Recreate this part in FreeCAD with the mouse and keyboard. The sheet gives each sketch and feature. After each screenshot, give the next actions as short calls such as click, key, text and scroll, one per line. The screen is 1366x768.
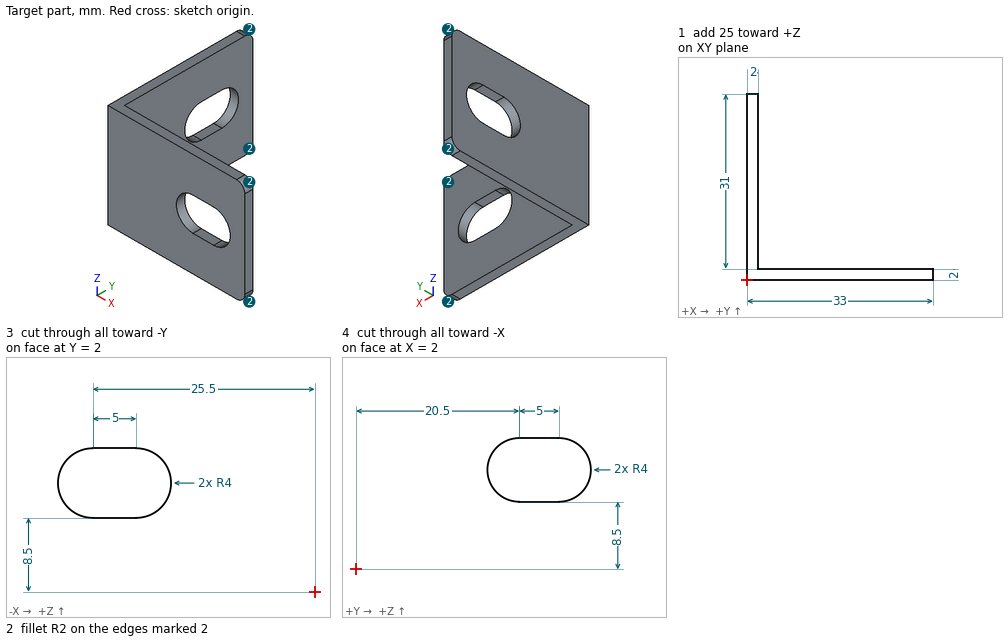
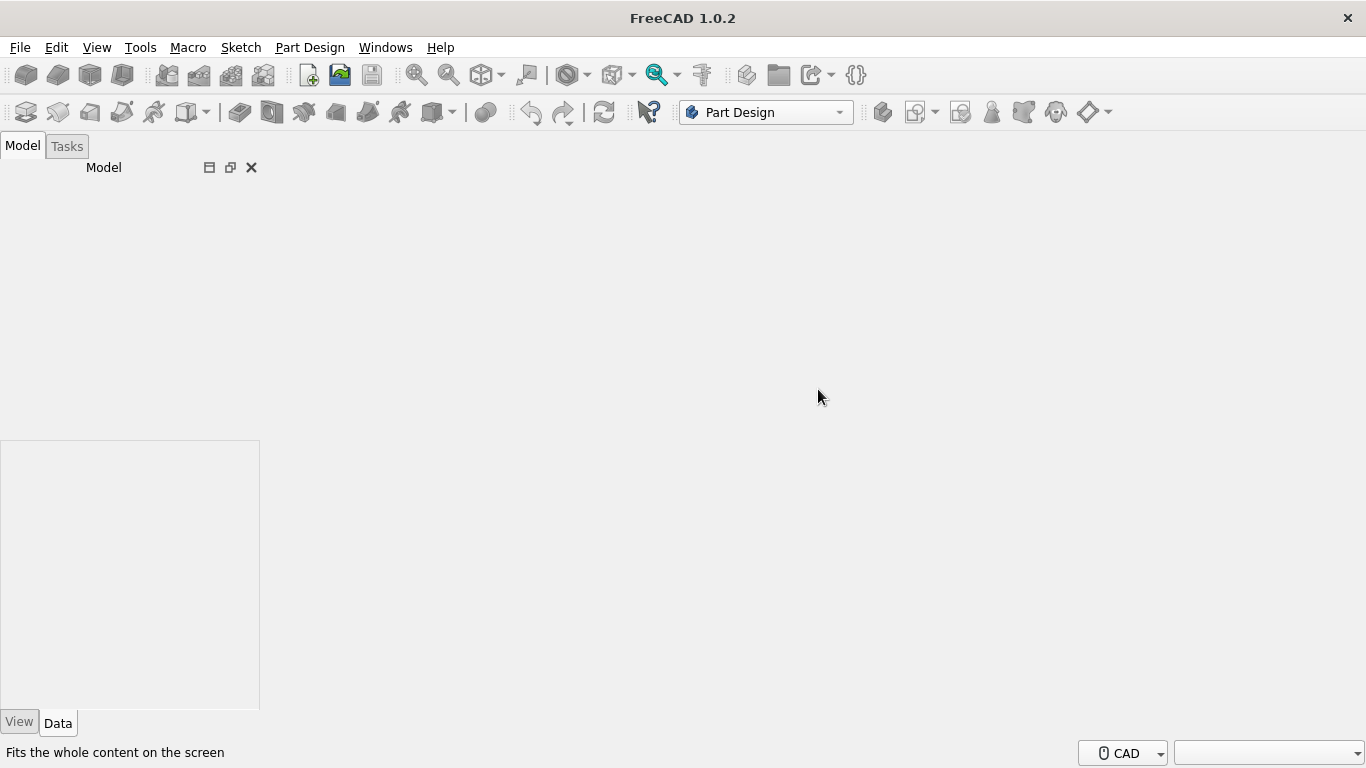
key(ctrl+n)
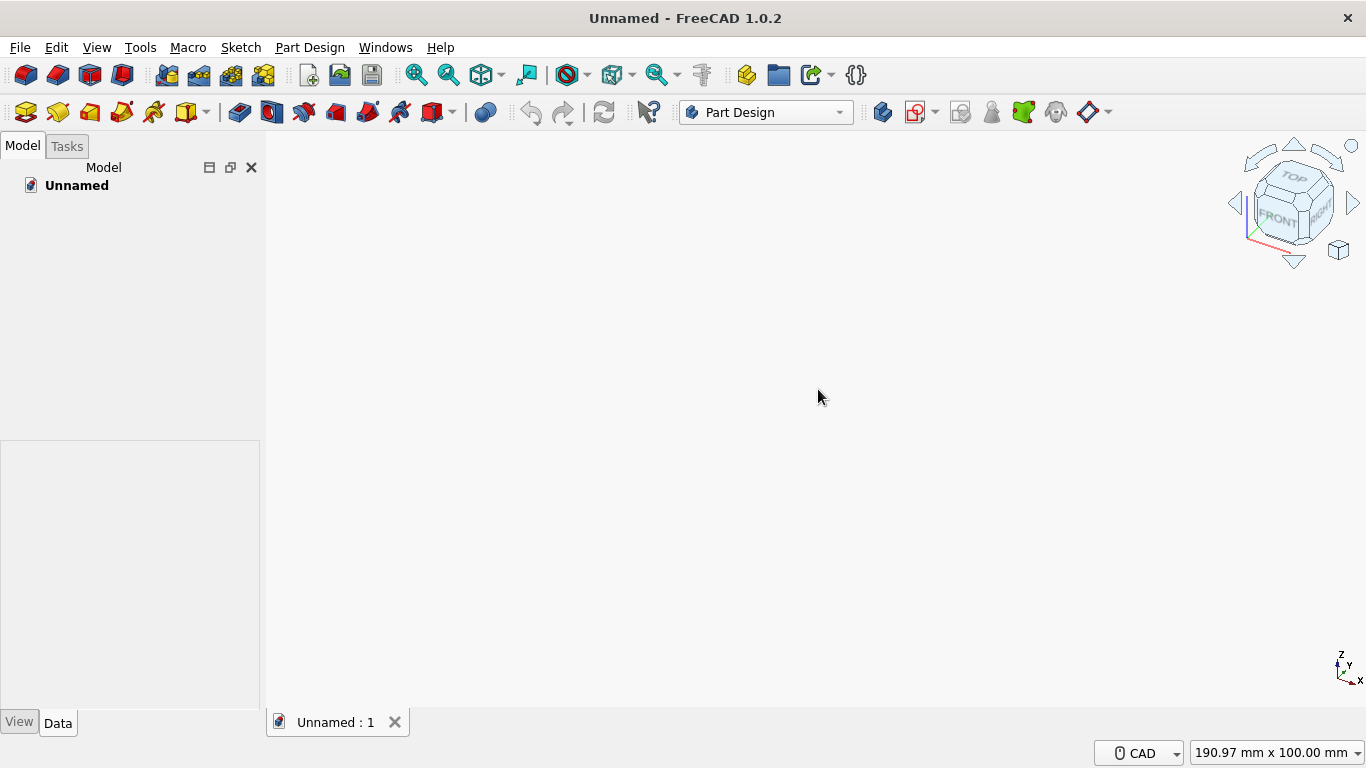
click(916, 112)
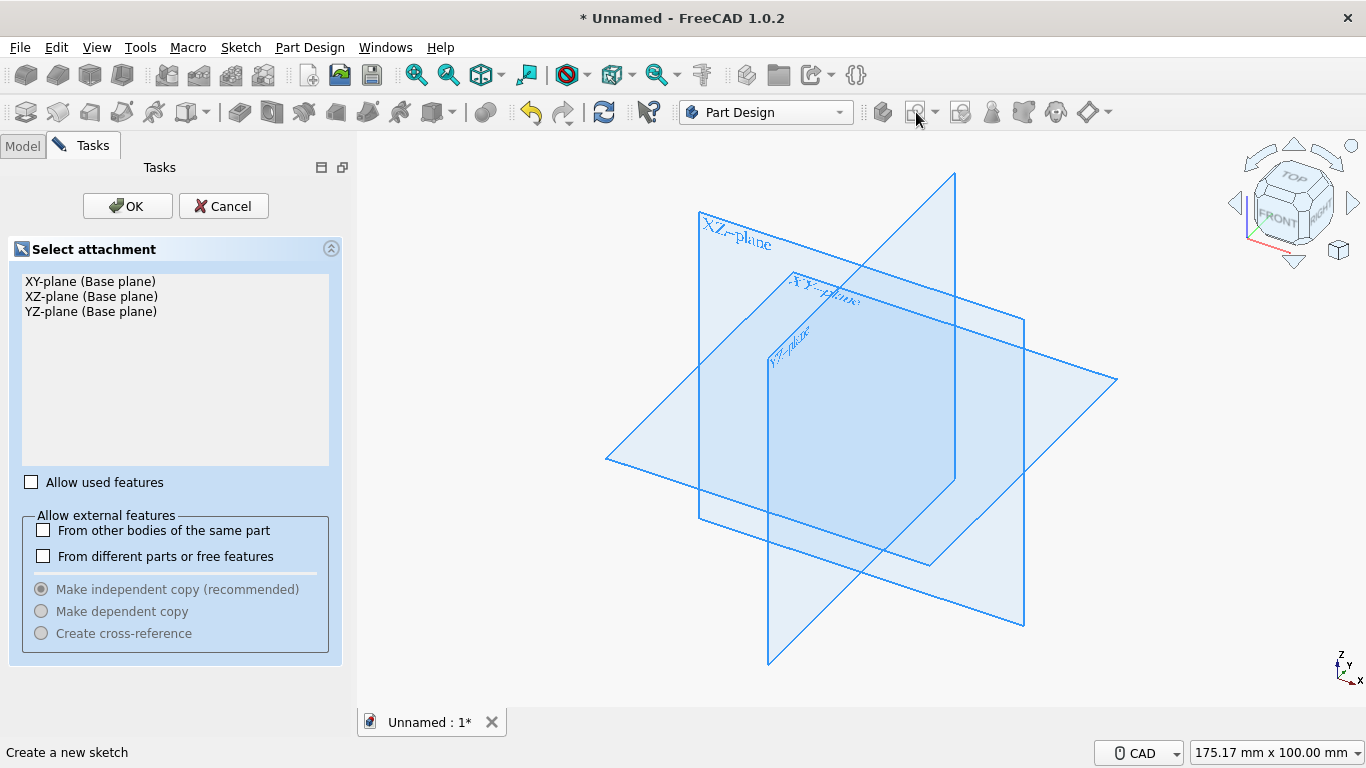
click(82, 282)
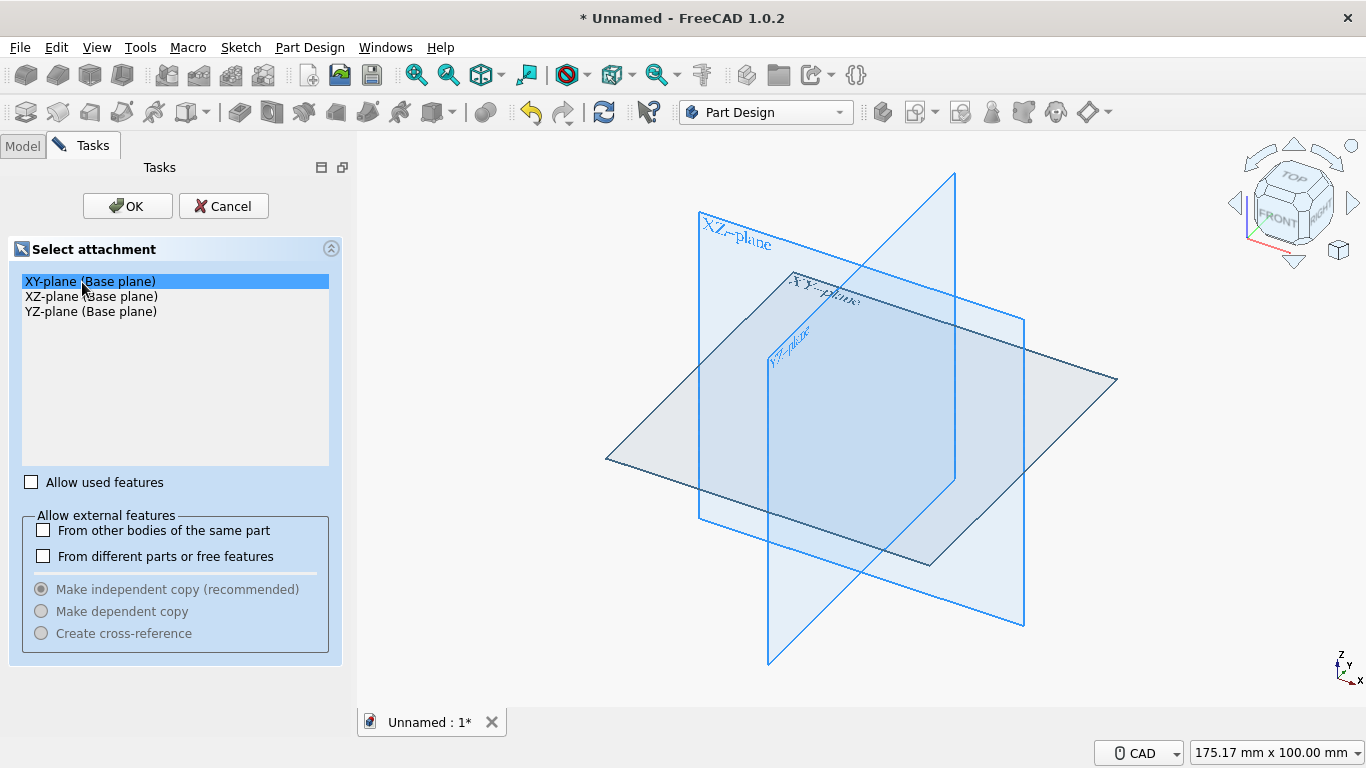
click(128, 206)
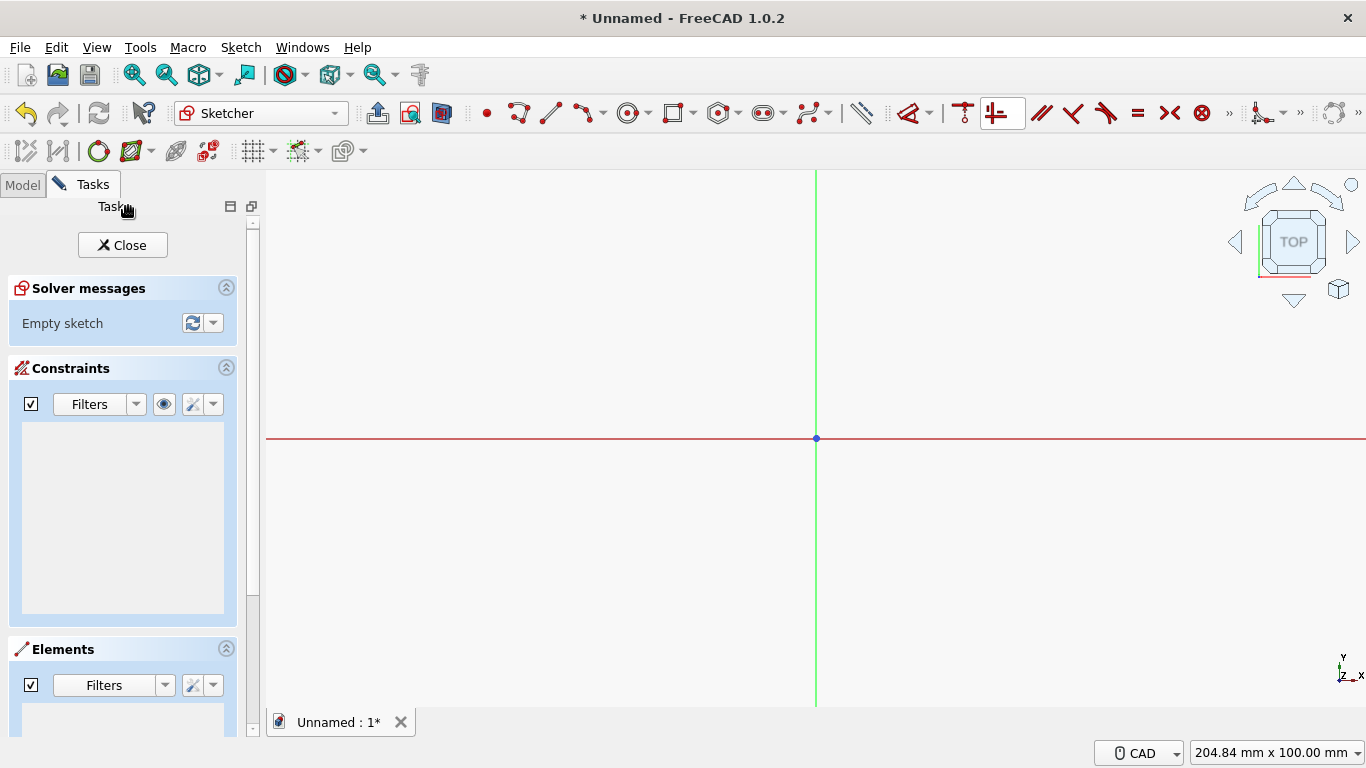
scroll(1096, 242, up, 3)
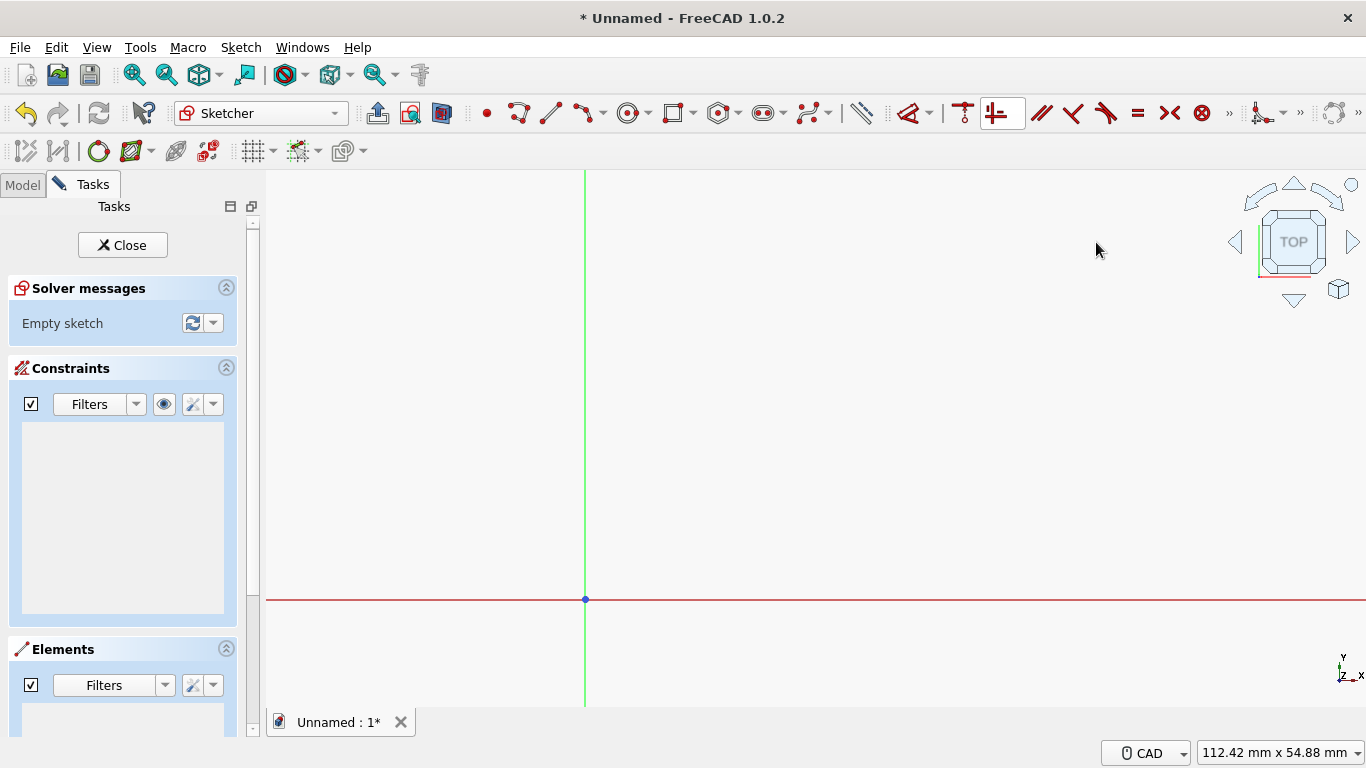
key(g)
key(m)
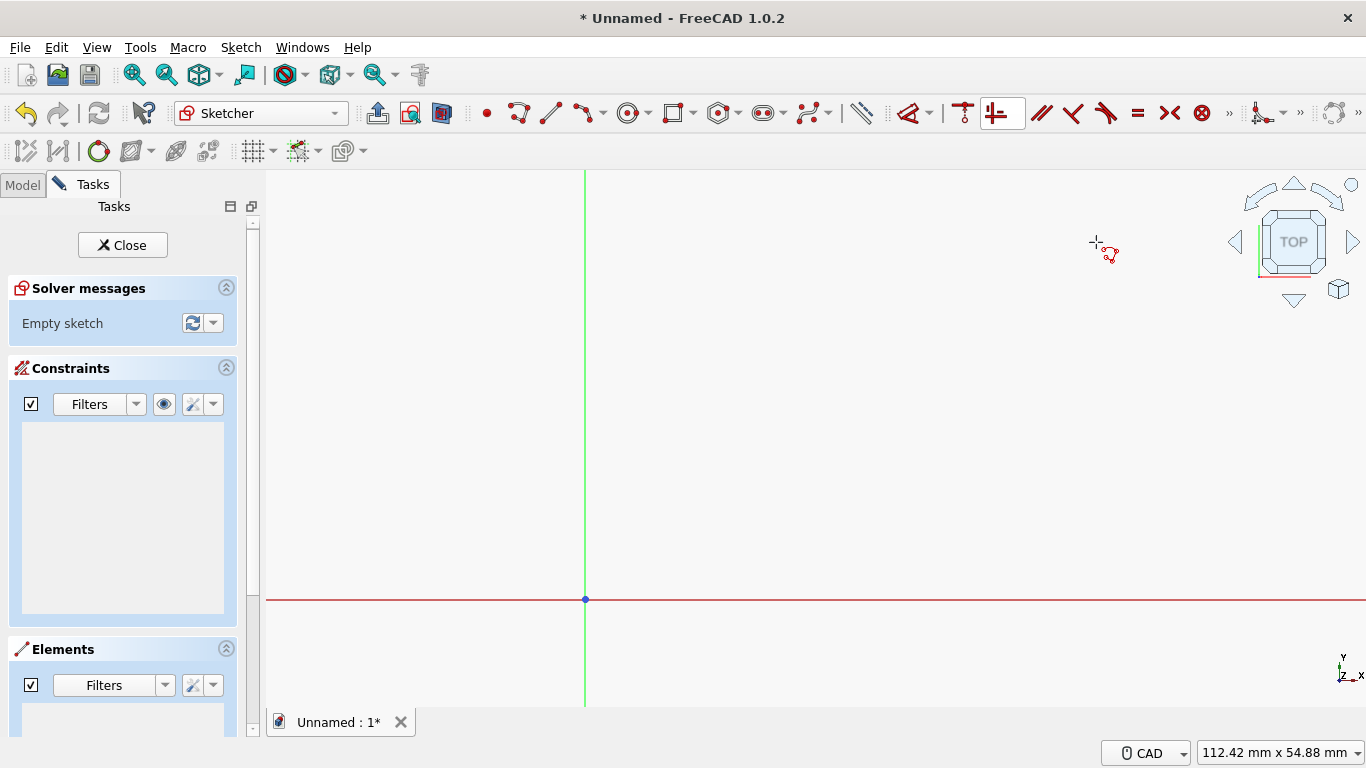
click(585, 600)
click(908, 591)
click(908, 580)
click(605, 580)
click(605, 277)
click(594, 277)
click(585, 600)
key(Escape)
key(Escape)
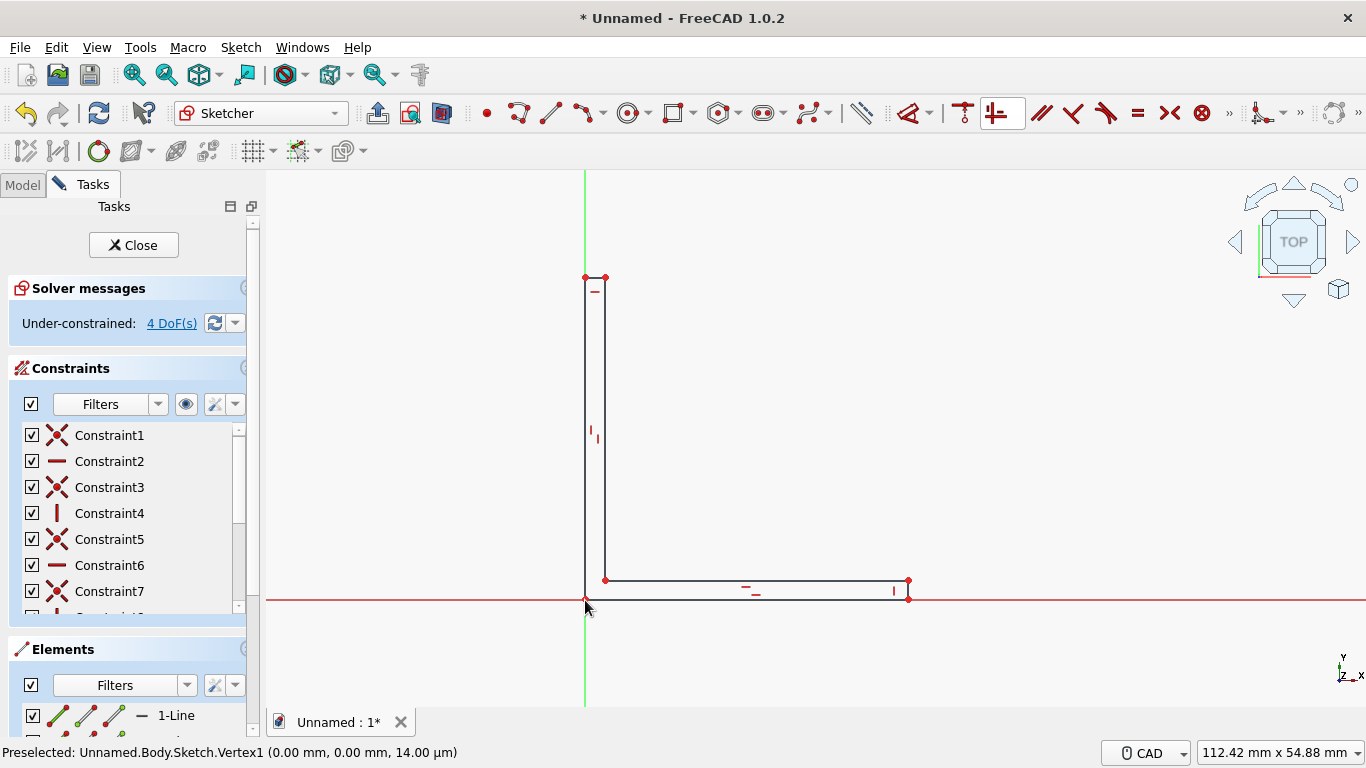
scroll(908, 590, up, 4)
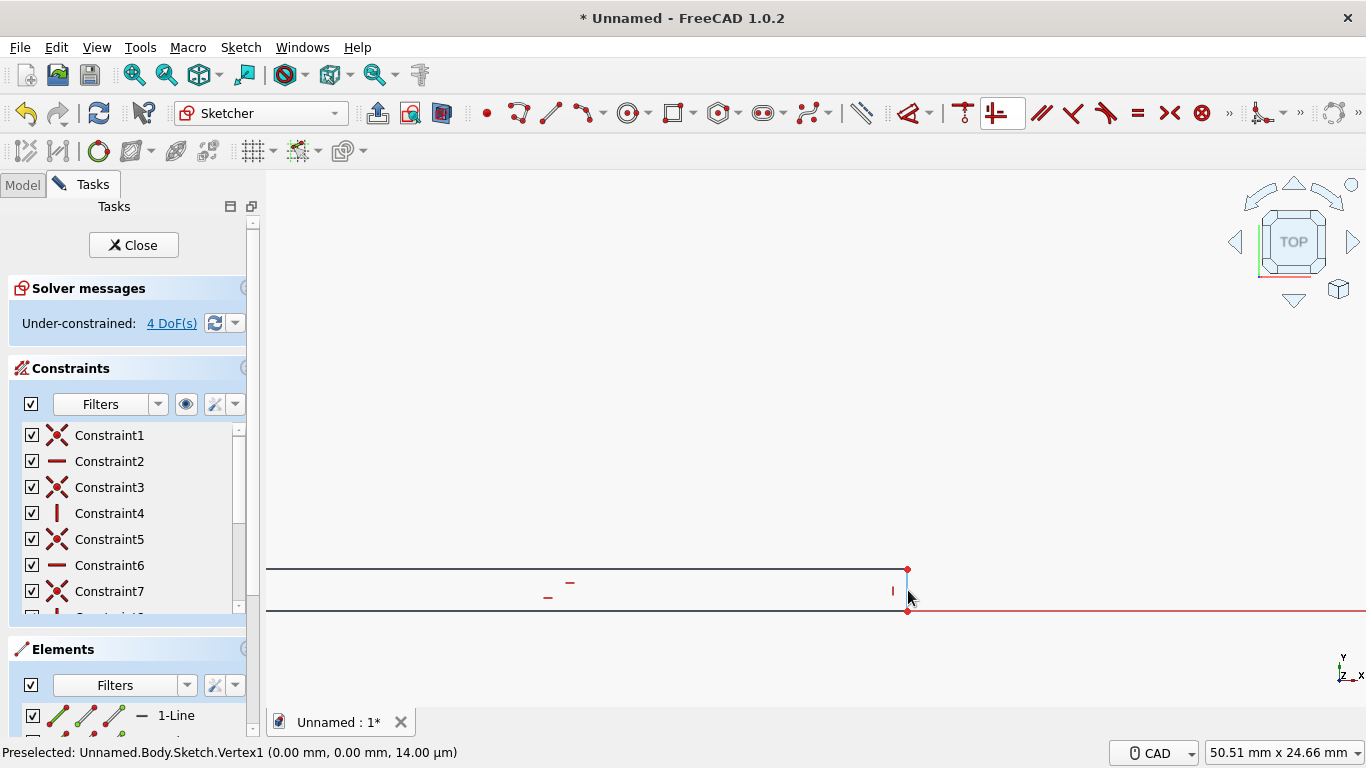
click(907, 590)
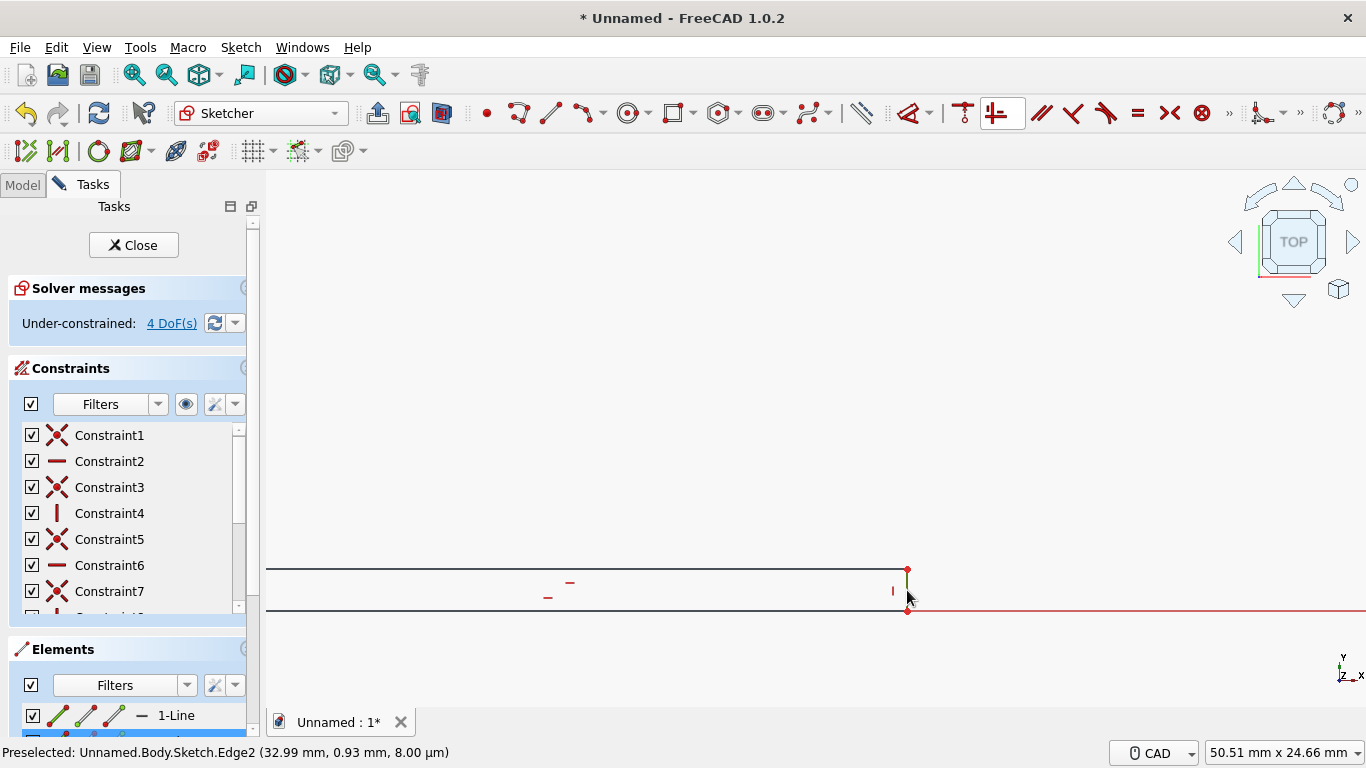
key(i)